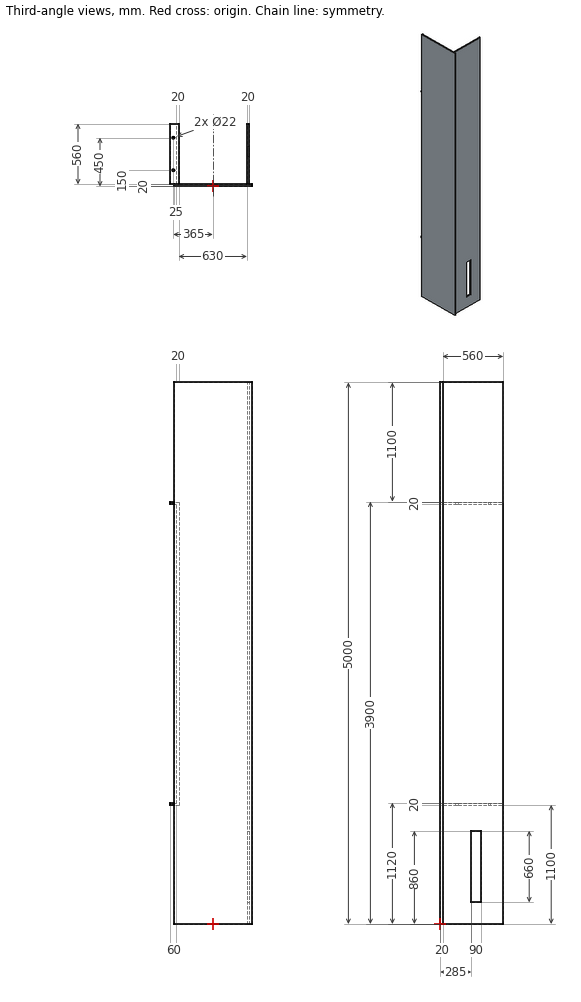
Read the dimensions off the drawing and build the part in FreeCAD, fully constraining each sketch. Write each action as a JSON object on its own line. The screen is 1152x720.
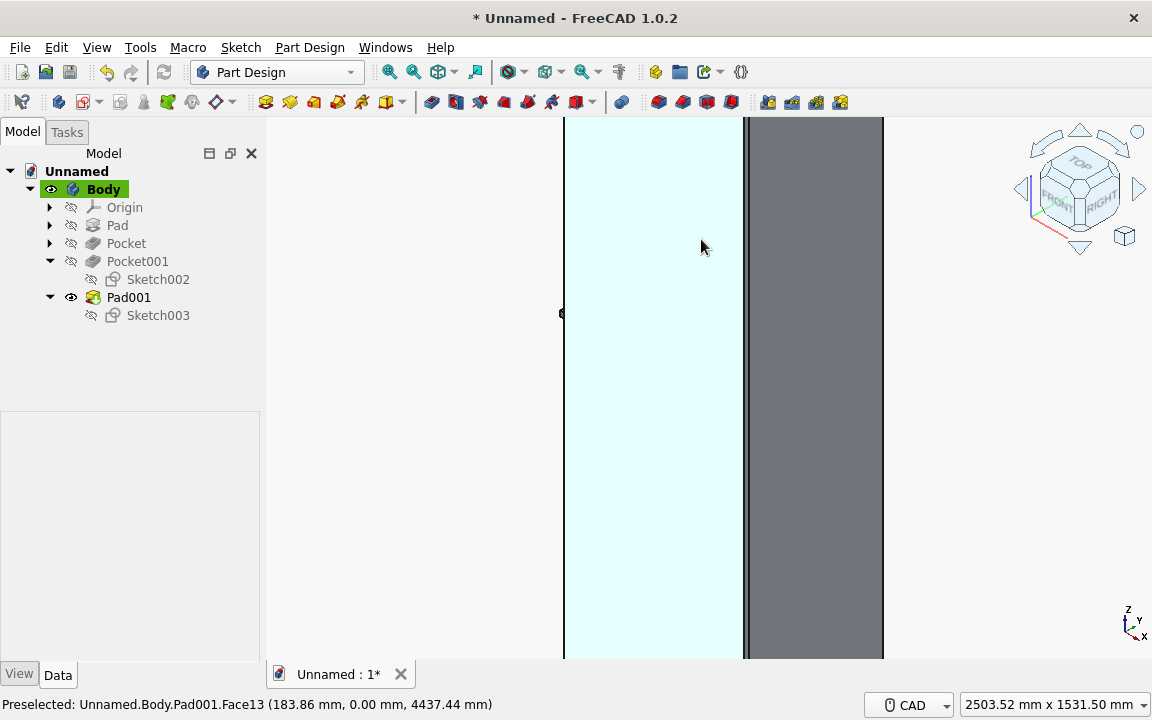
{"action": "left_click", "coordinate": [390, 72]}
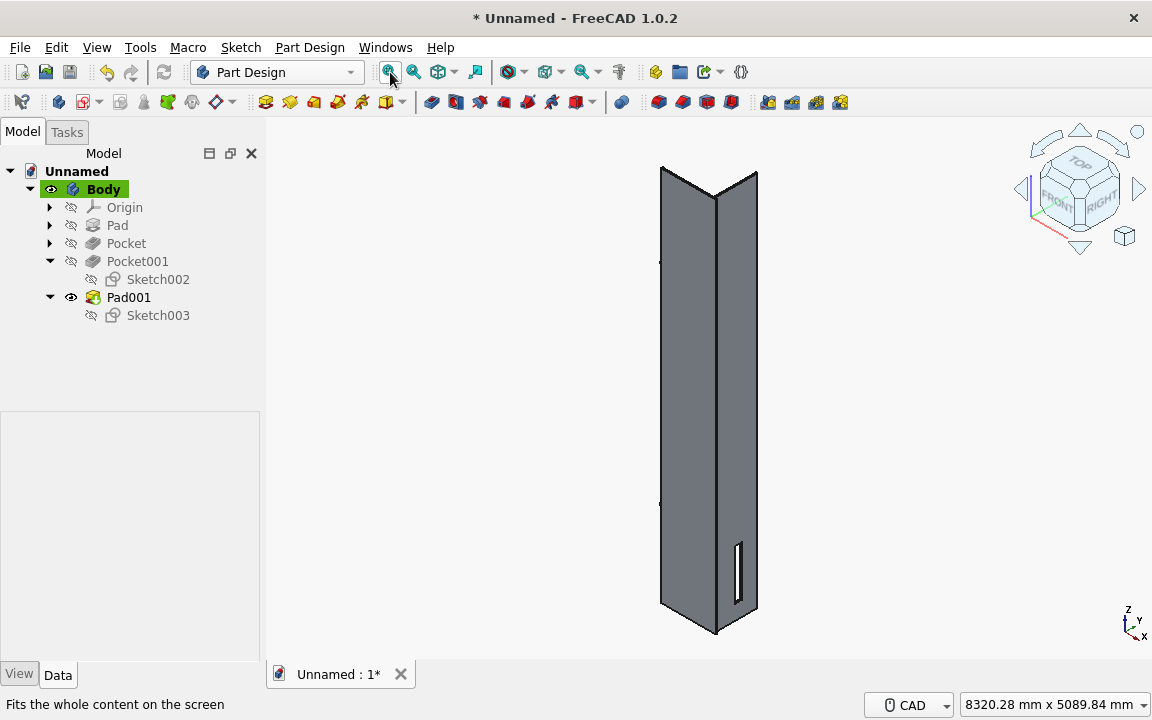
{"action": "key", "text": "2"}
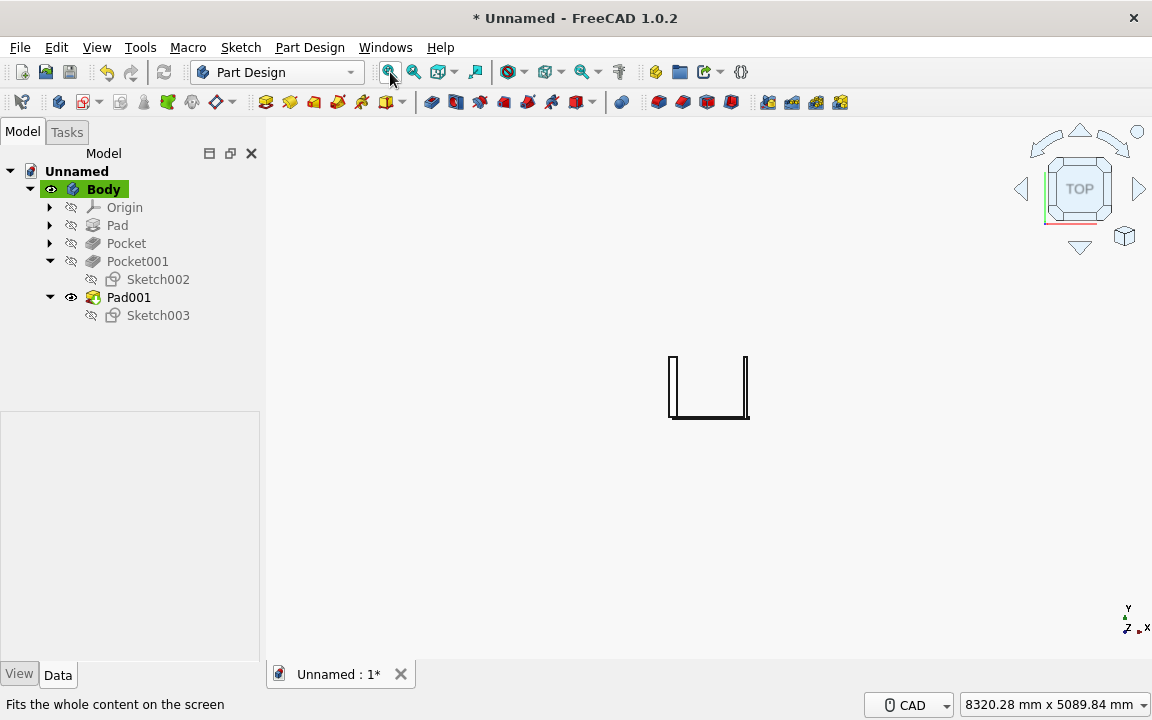
{"action": "left_click", "coordinate": [390, 72]}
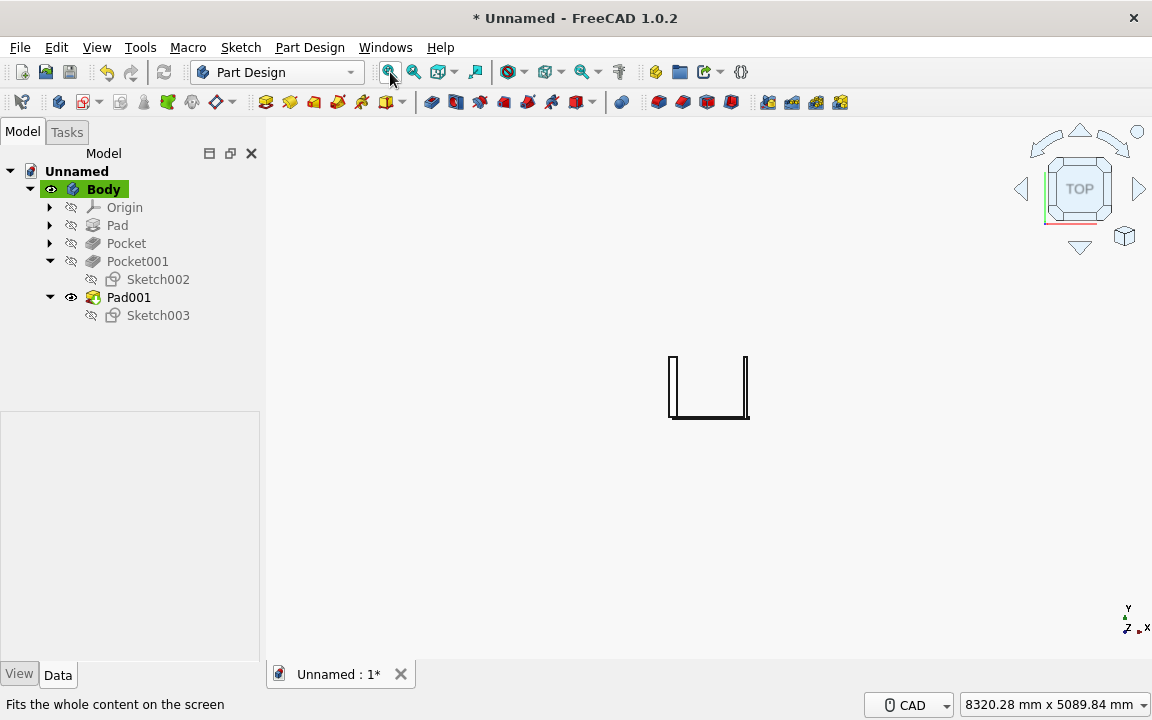
{"action": "scroll", "coordinate": [673, 360], "scroll_direction": "up", "scroll_amount": 6}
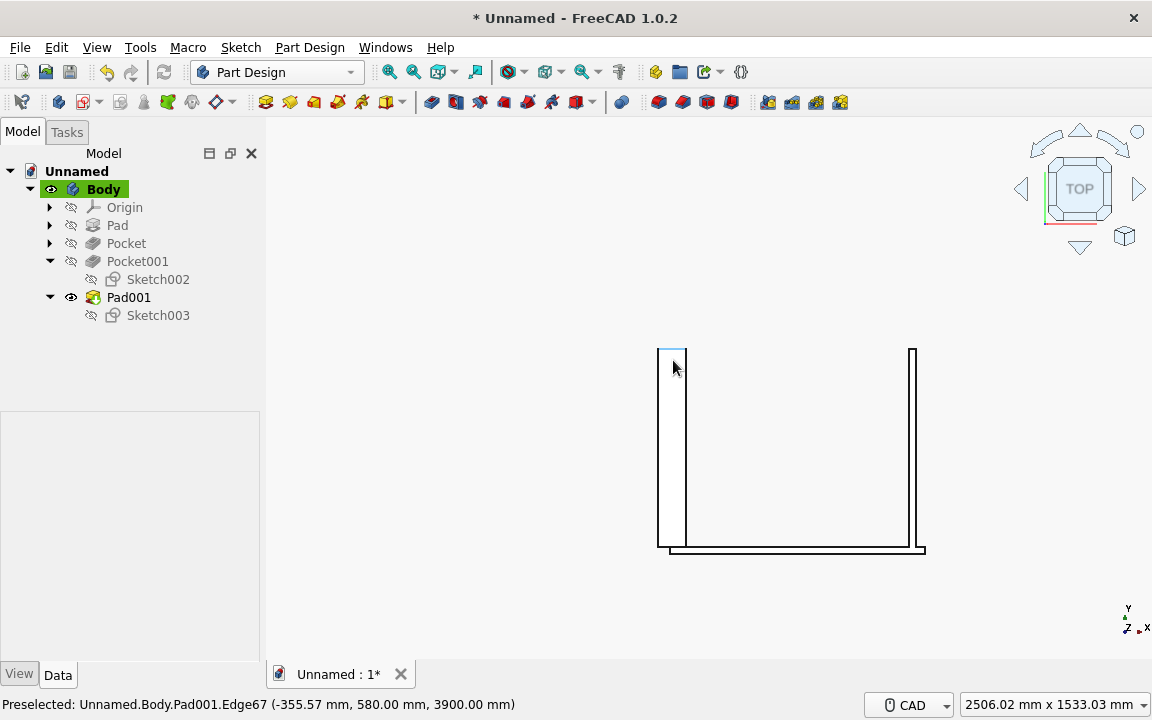
{"action": "left_click", "coordinate": [672, 363]}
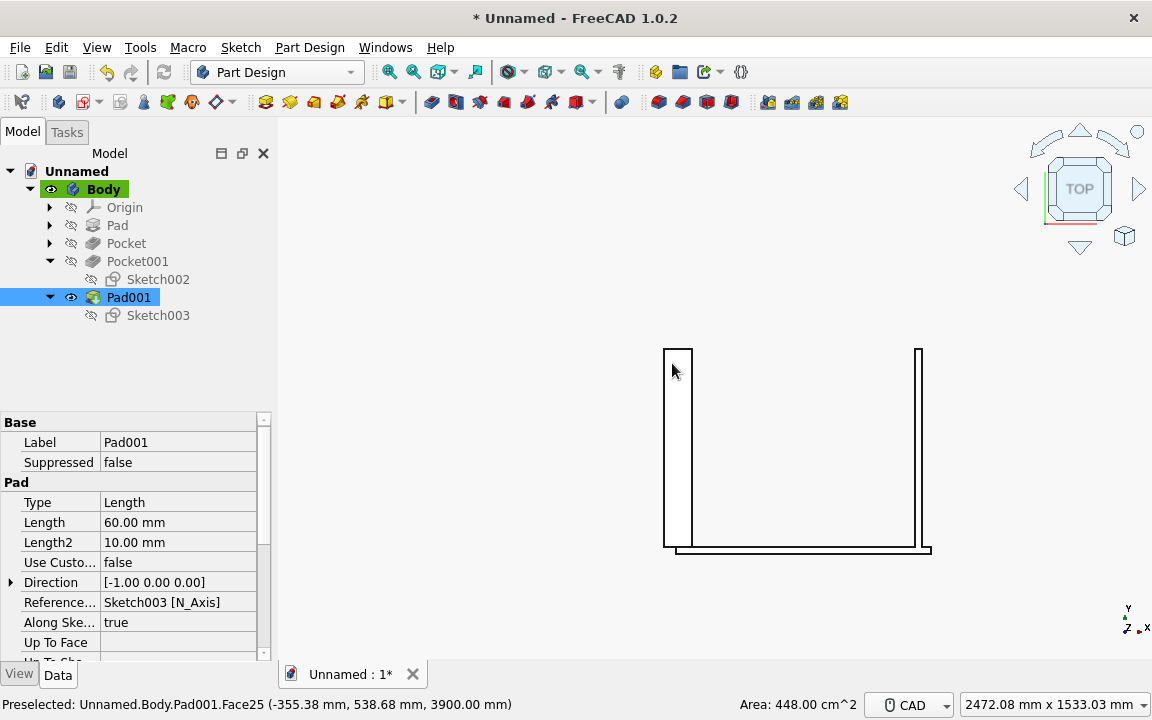
{"action": "left_click", "coordinate": [84, 102]}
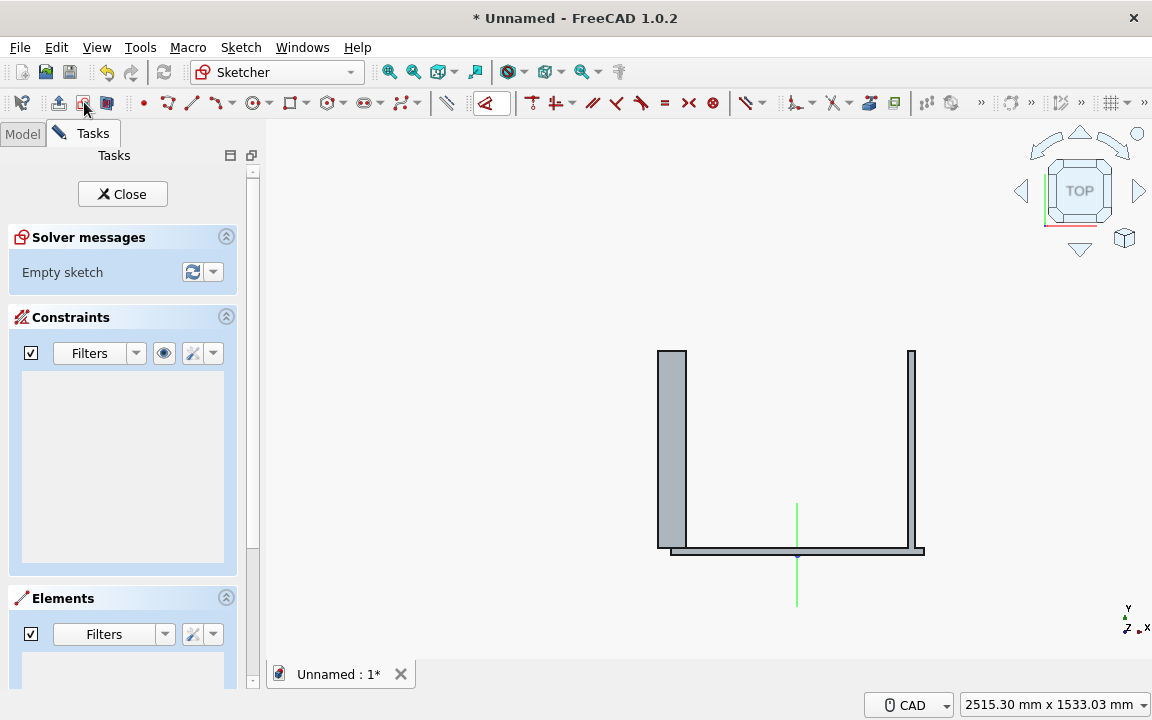
{"action": "left_click", "coordinate": [108, 104]}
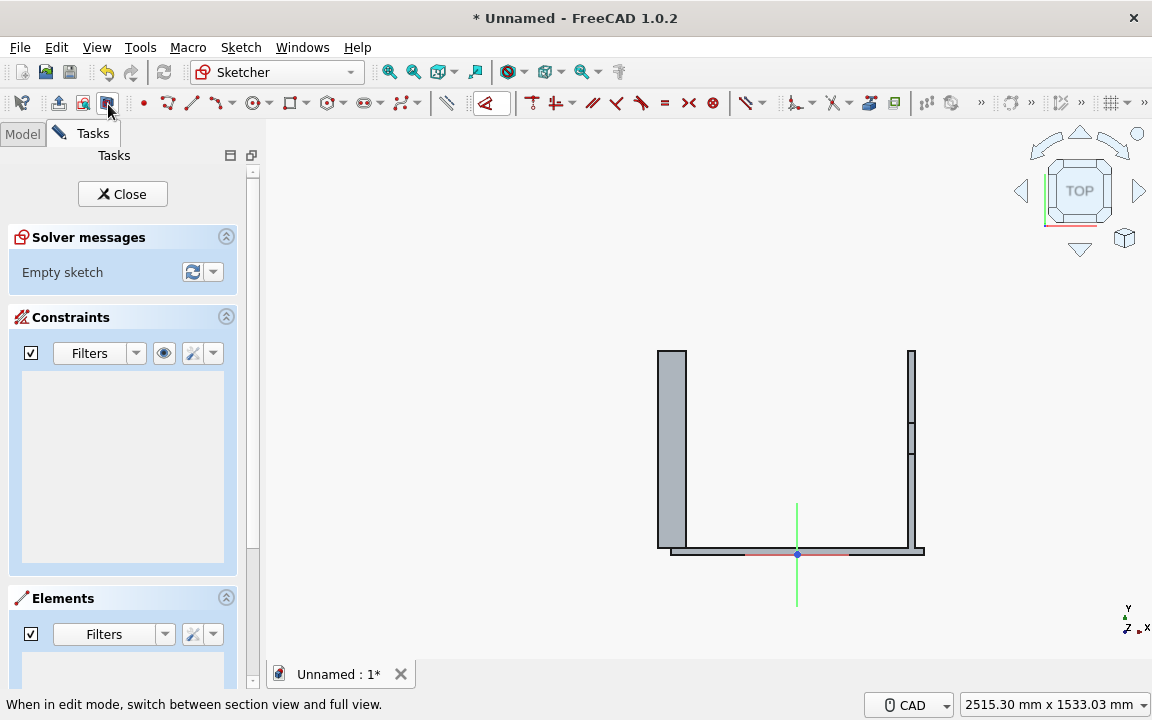
{"action": "scroll", "coordinate": [805, 543], "scroll_direction": "up", "scroll_amount": 4}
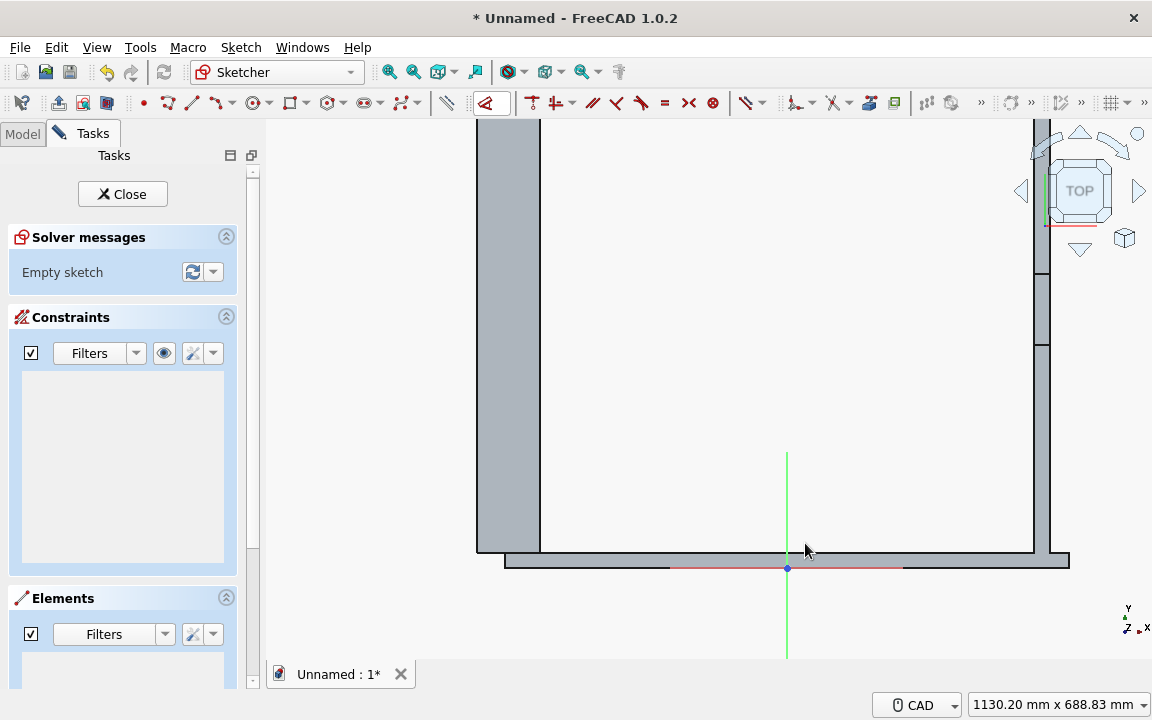
{"action": "left_click", "coordinate": [254, 104]}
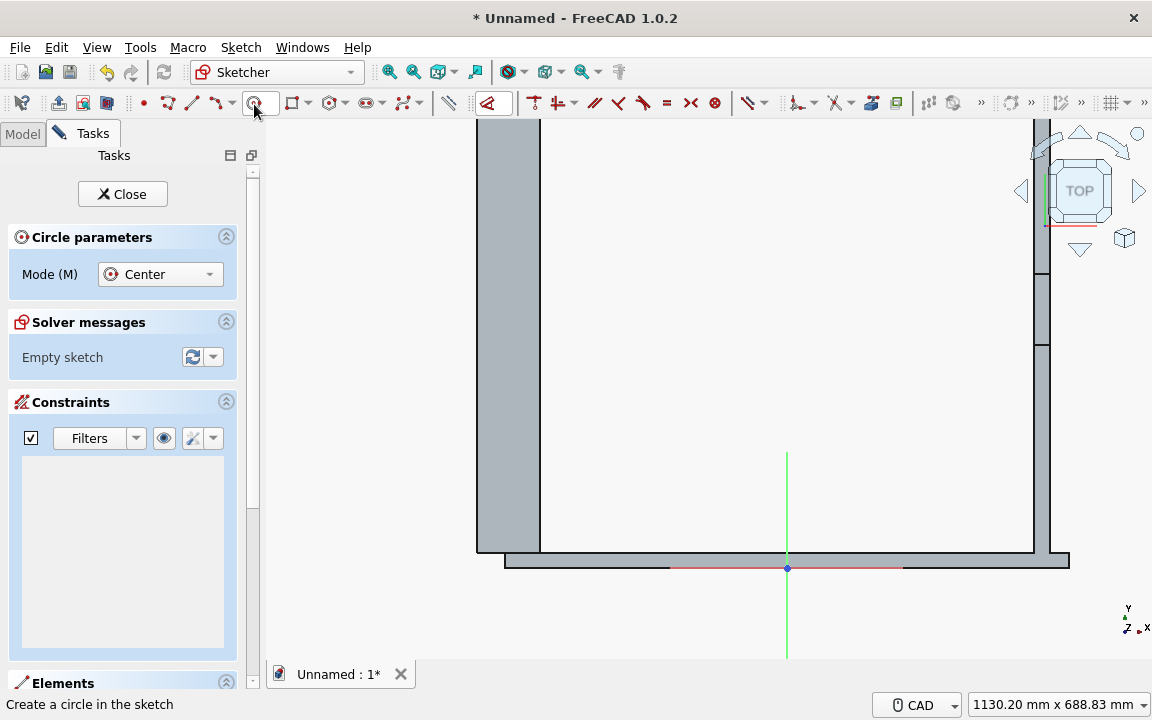
{"action": "scroll", "coordinate": [501, 216], "scroll_direction": "up", "scroll_amount": 5}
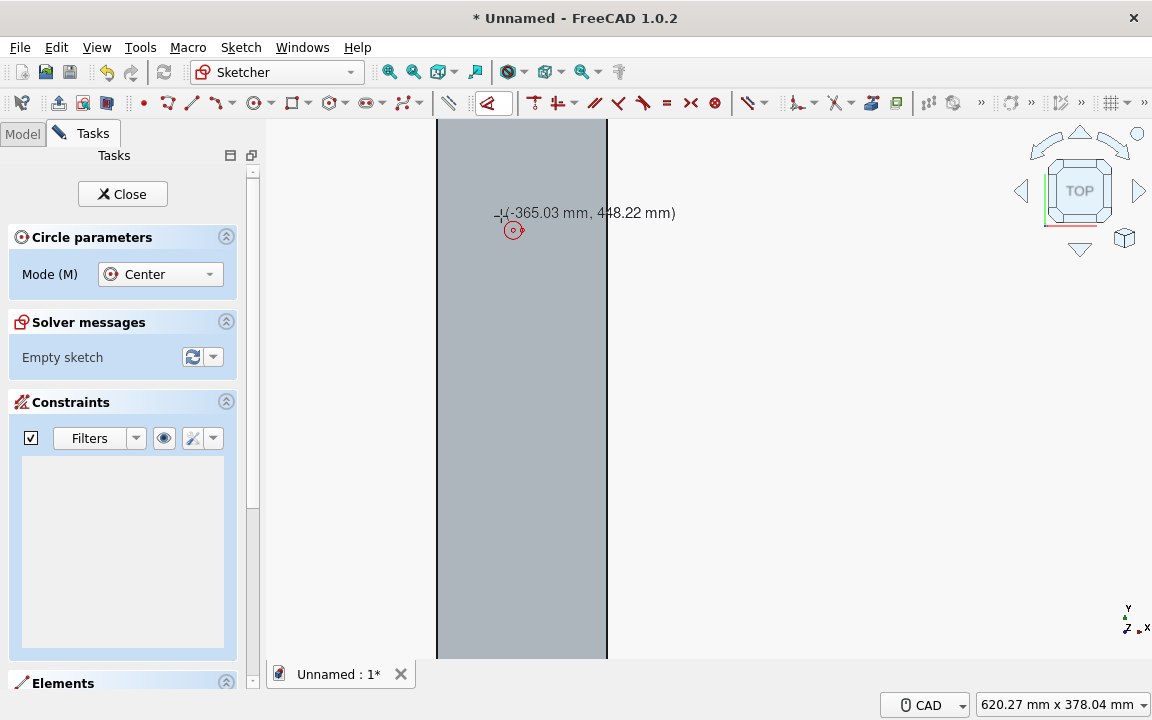
{"action": "left_click", "coordinate": [501, 215]}
{"action": "mouse_move", "coordinate": [517, 198]}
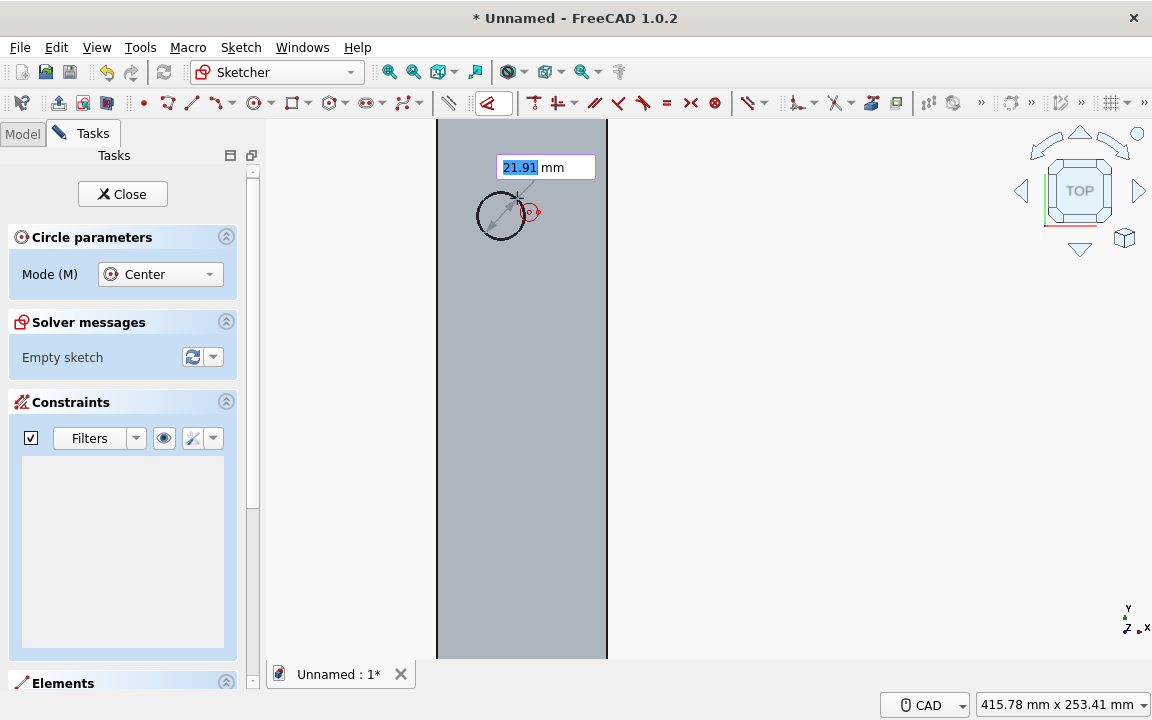
{"action": "type", "text": "22"}
{"action": "key", "text": "Return"}